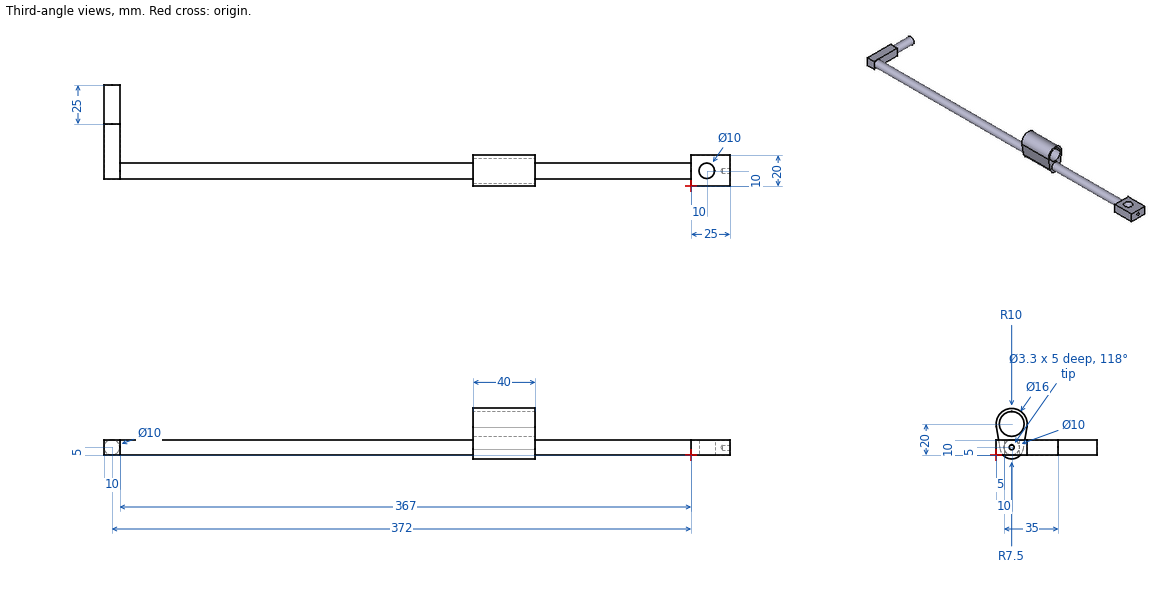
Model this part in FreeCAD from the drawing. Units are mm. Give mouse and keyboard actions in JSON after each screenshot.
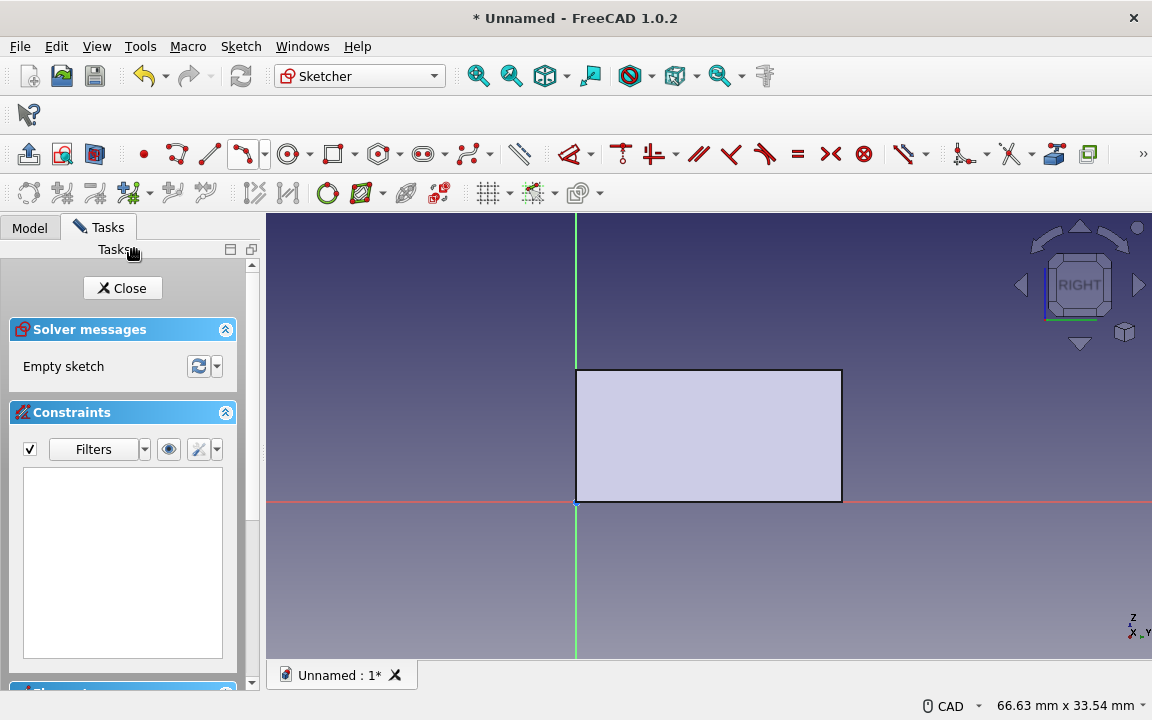
{"action": "key", "text": "q s"}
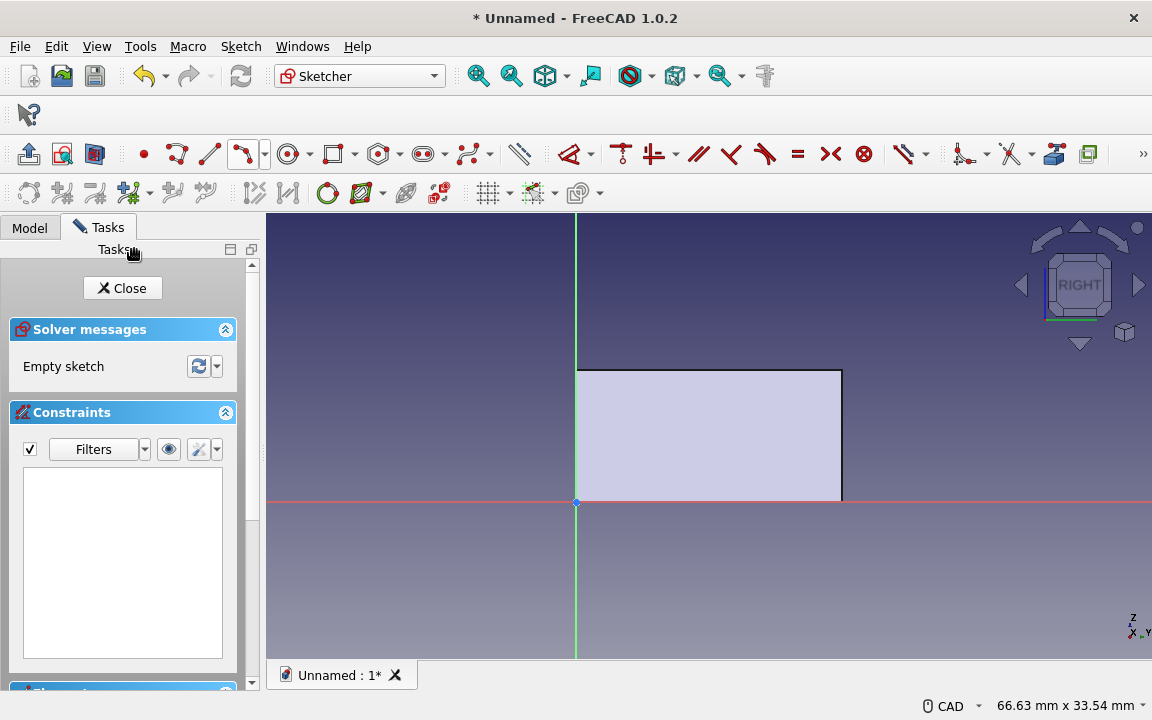
{"action": "scroll", "coordinate": [705, 436], "scroll_direction": "up", "scroll_amount": 4}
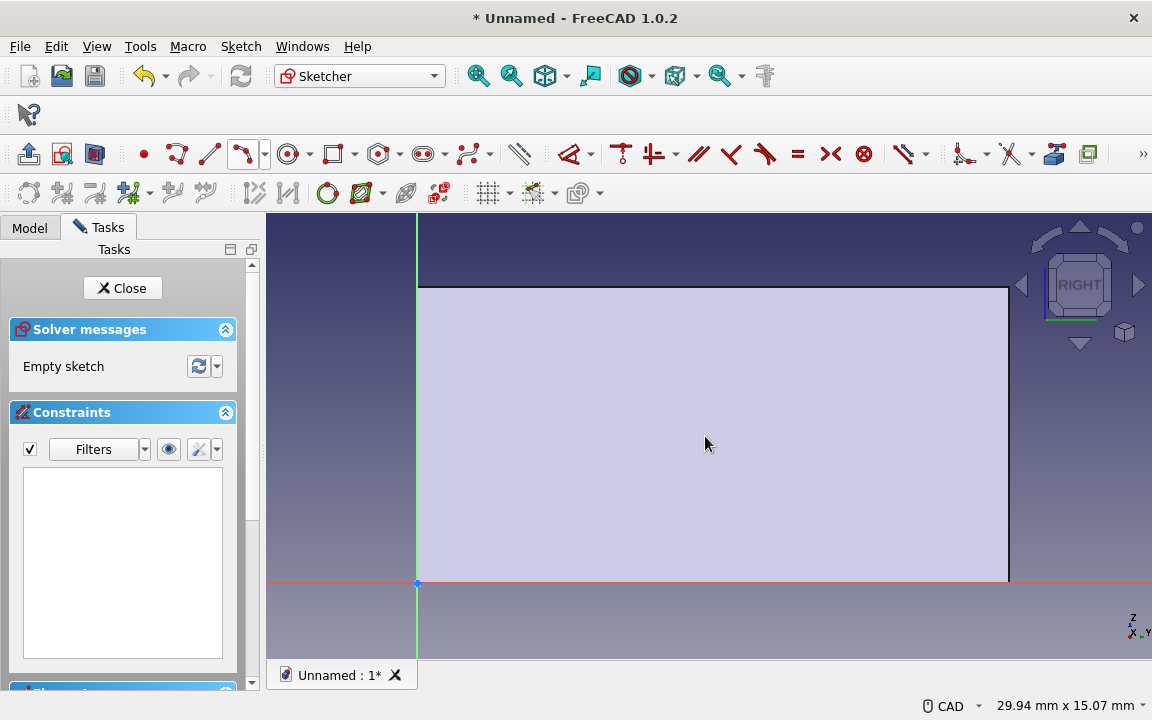
{"action": "key", "text": "g c"}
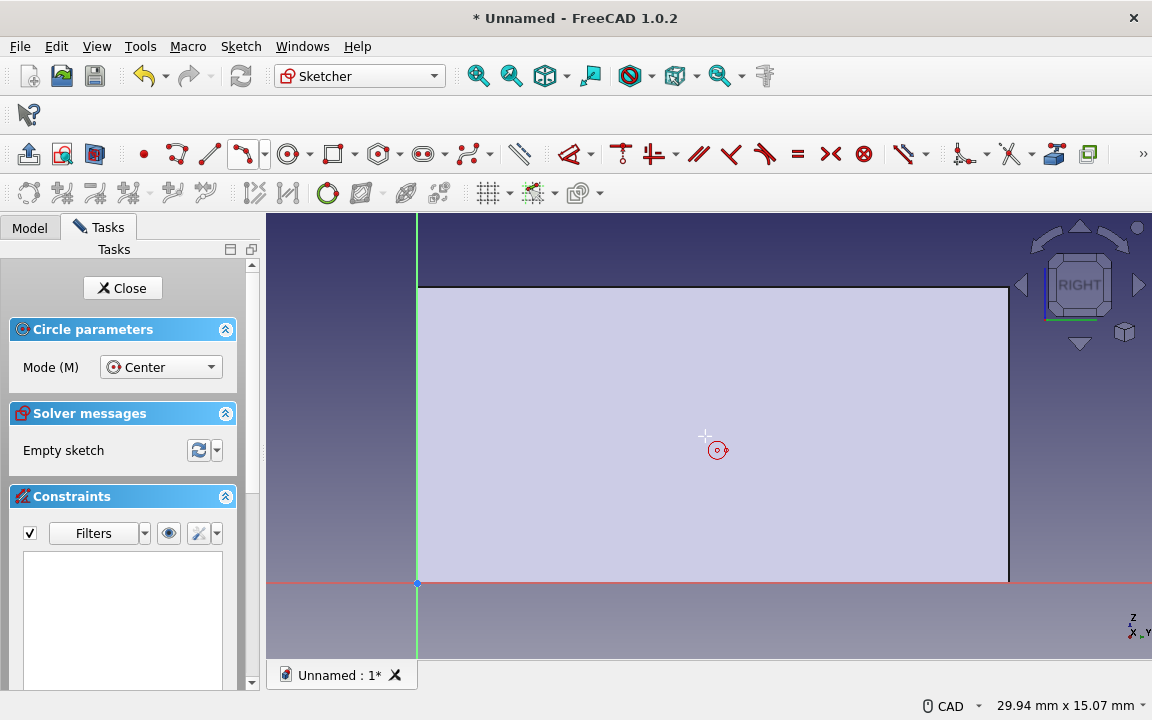
{"action": "left_click", "coordinate": [713, 435]}
{"action": "mouse_move", "coordinate": [818, 331]}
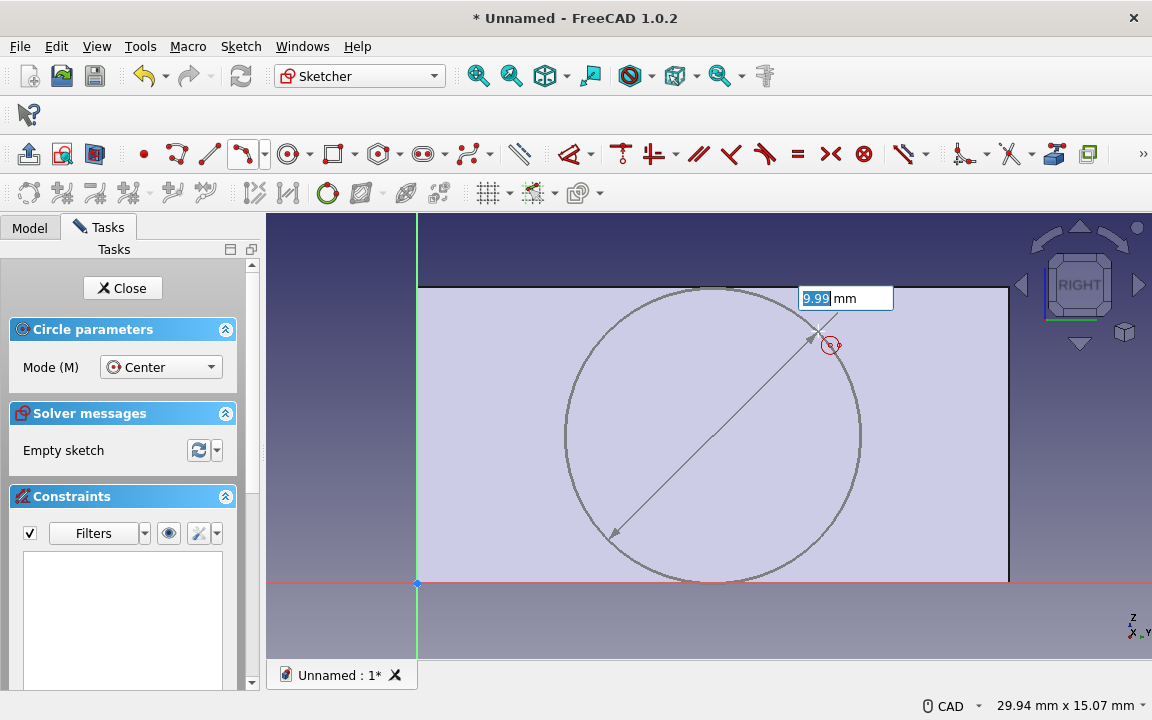
{"action": "type", "text": "10"}
{"action": "key", "text": "Return"}
{"action": "key", "text": "Escape"}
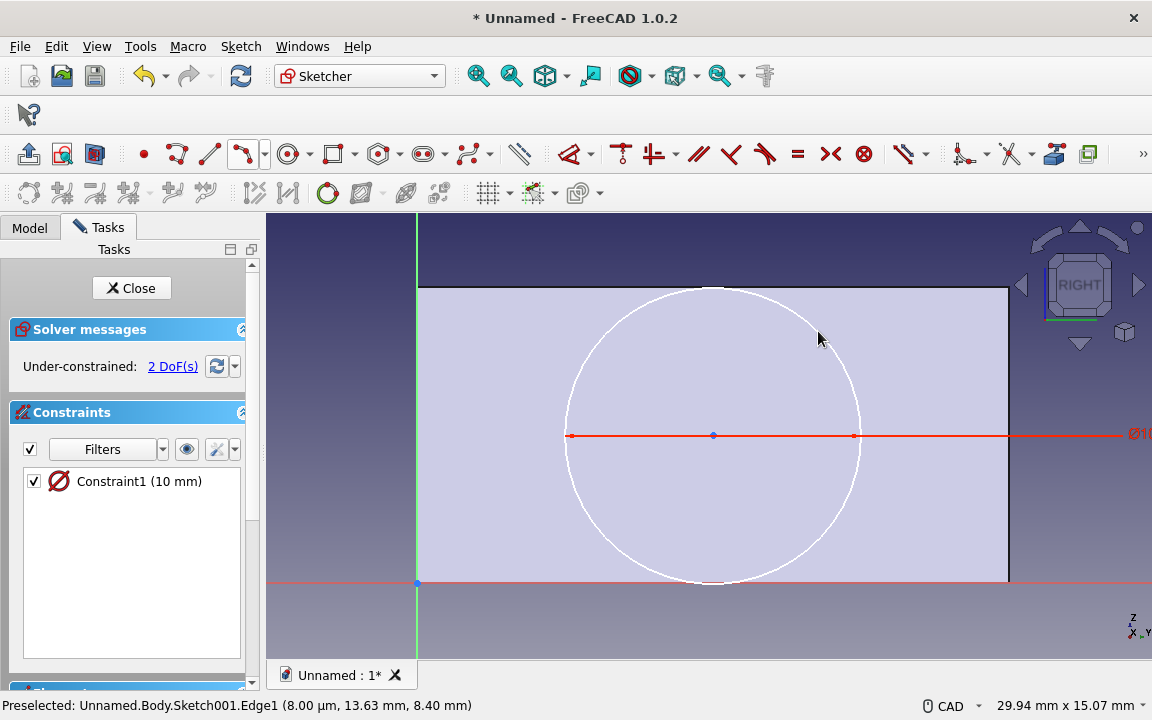
{"action": "left_click", "coordinate": [568, 154]}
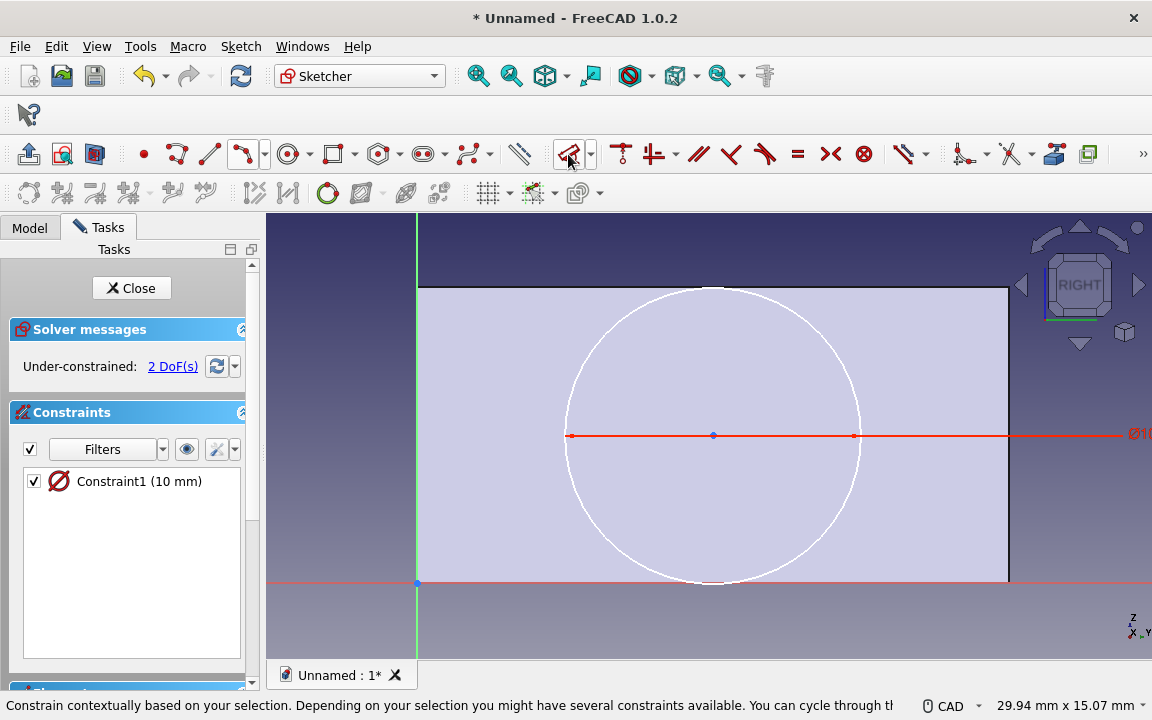
{"action": "left_click", "coordinate": [713, 436]}
{"action": "left_click", "coordinate": [383, 510]}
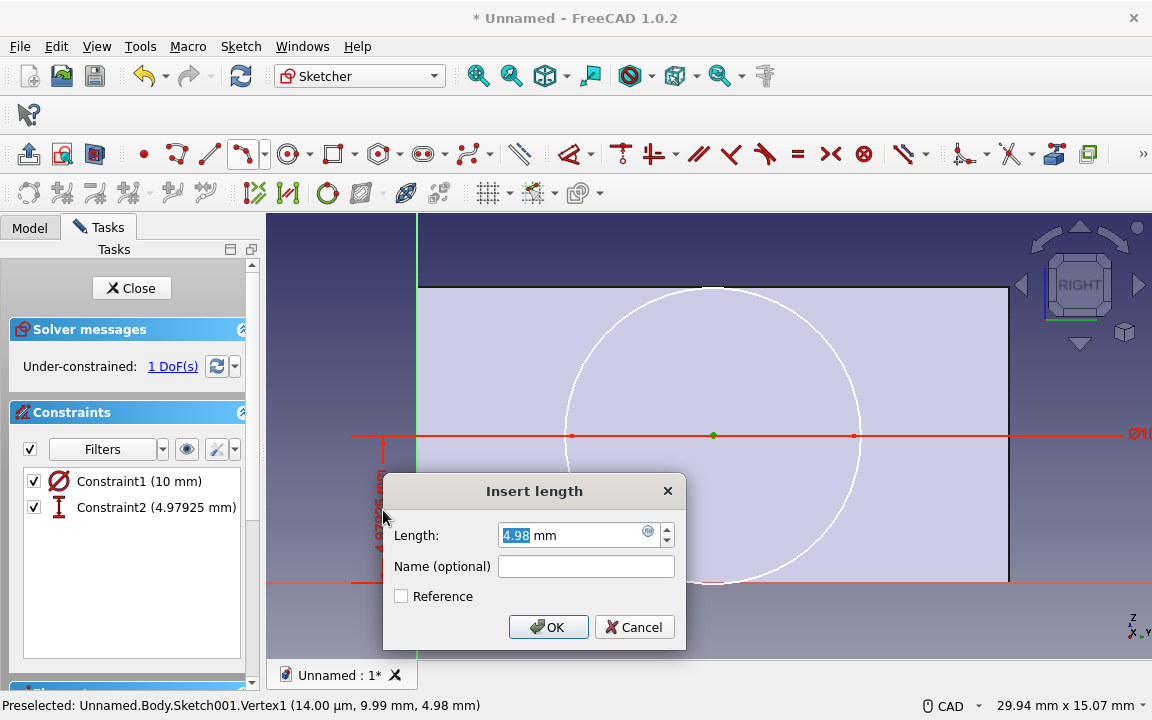
{"action": "type", "text": "5"}
{"action": "key", "text": "Return"}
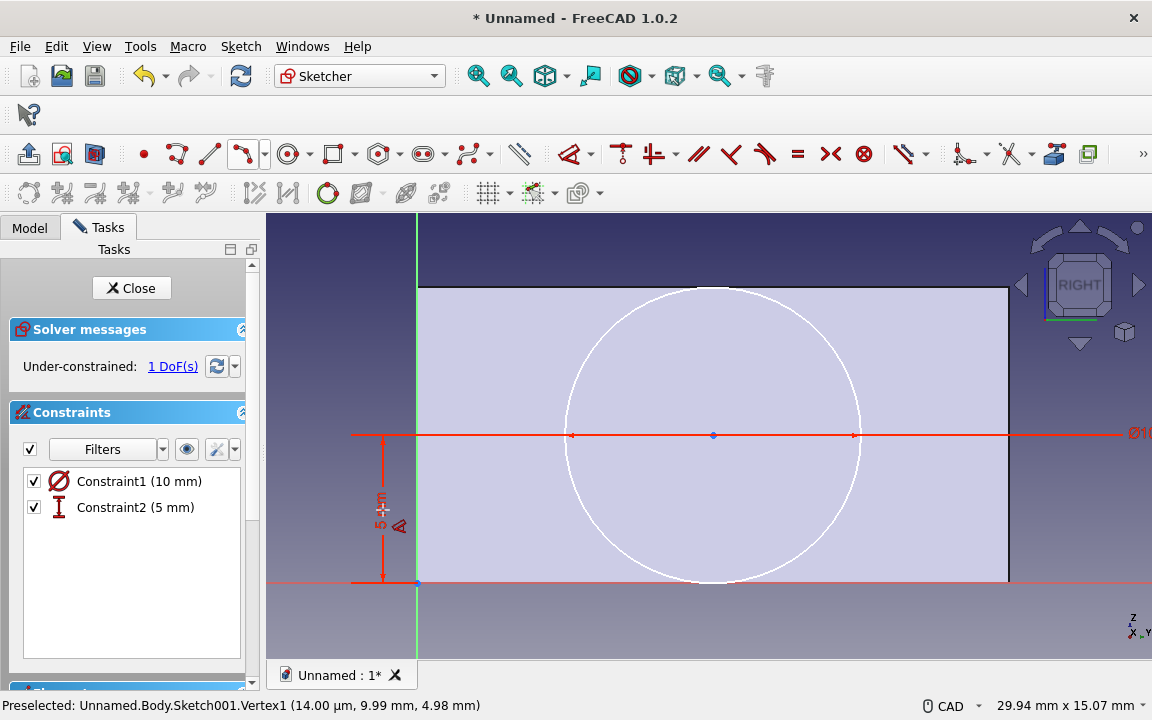
{"action": "left_click", "coordinate": [713, 435]}
{"action": "left_click", "coordinate": [565, 617]}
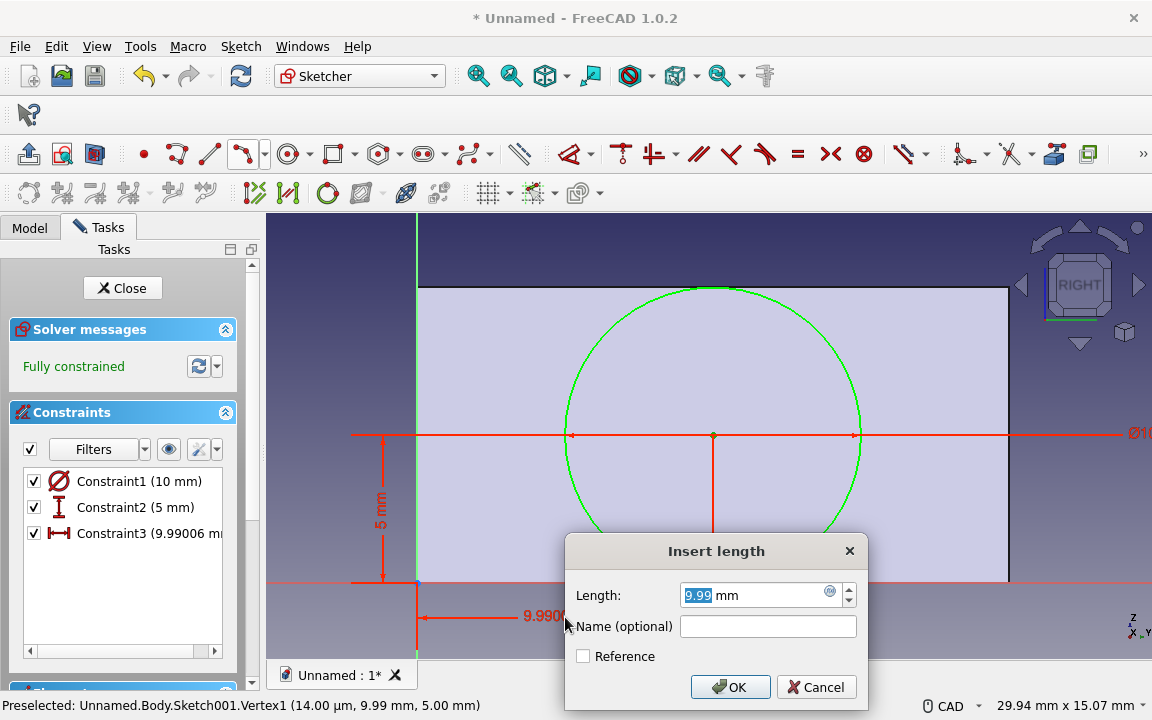
{"action": "type", "text": "10"}
{"action": "key", "text": "Return"}
{"action": "key", "text": "Escape"}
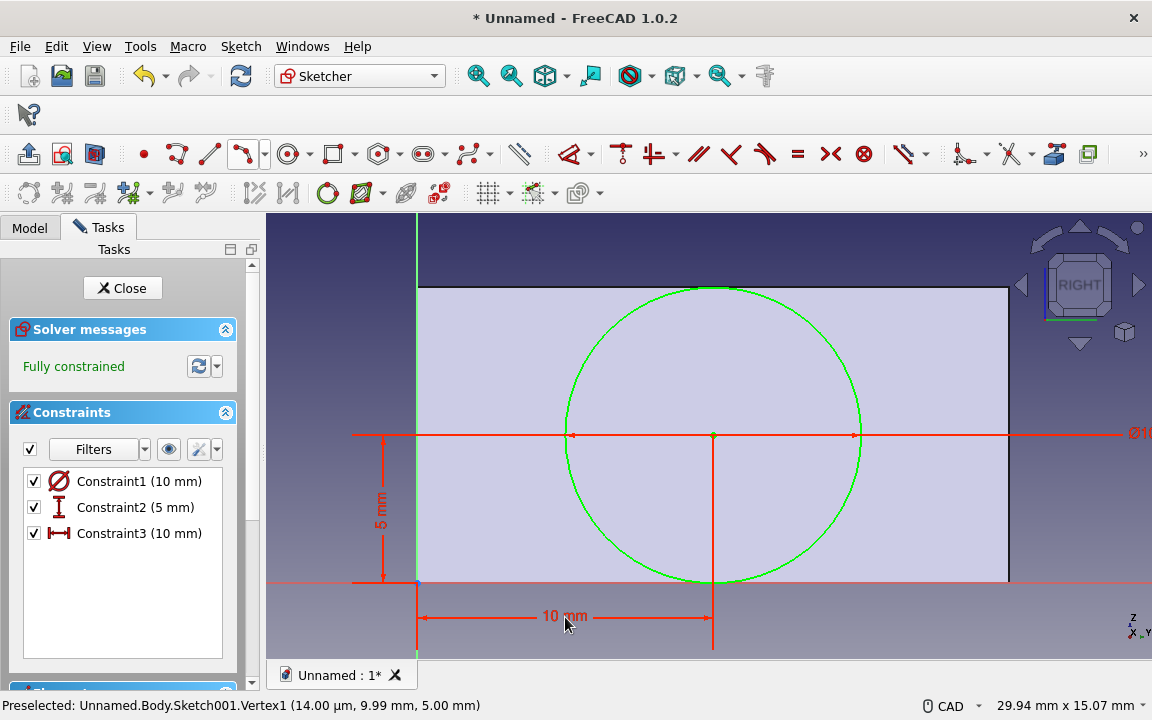
{"action": "left_click", "coordinate": [123, 288]}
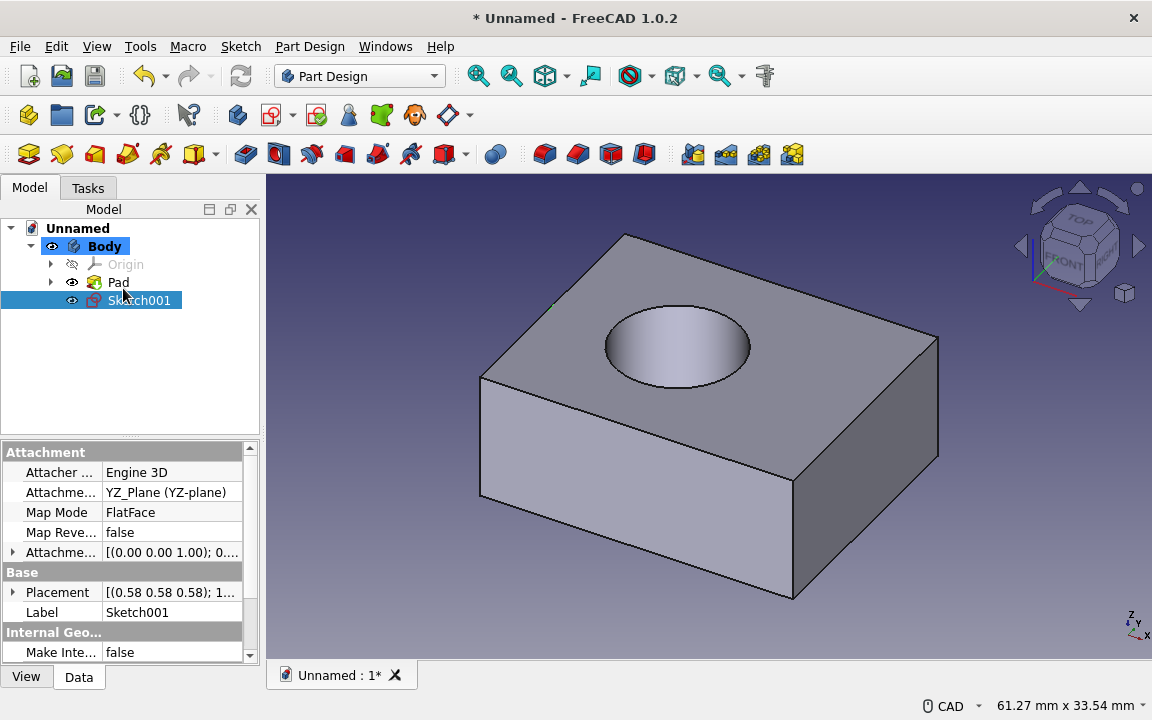
{"action": "left_click", "coordinate": [29, 154]}